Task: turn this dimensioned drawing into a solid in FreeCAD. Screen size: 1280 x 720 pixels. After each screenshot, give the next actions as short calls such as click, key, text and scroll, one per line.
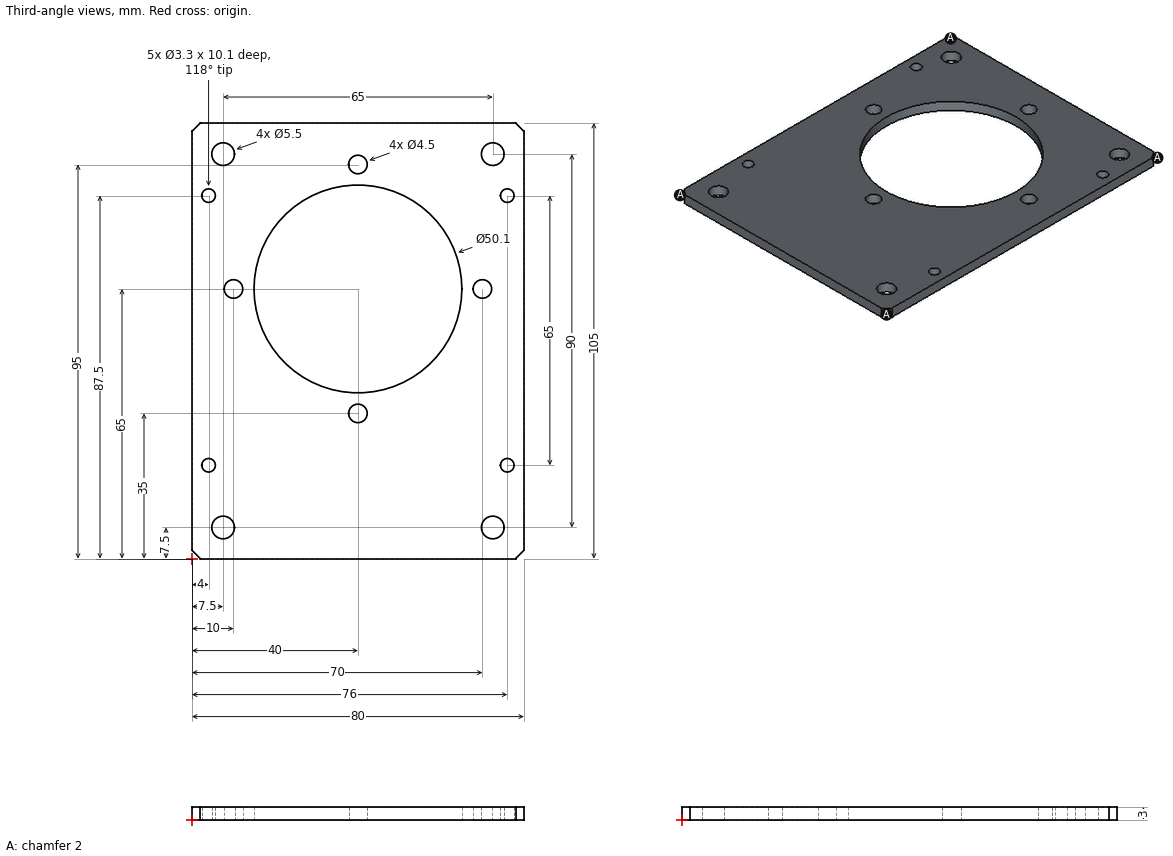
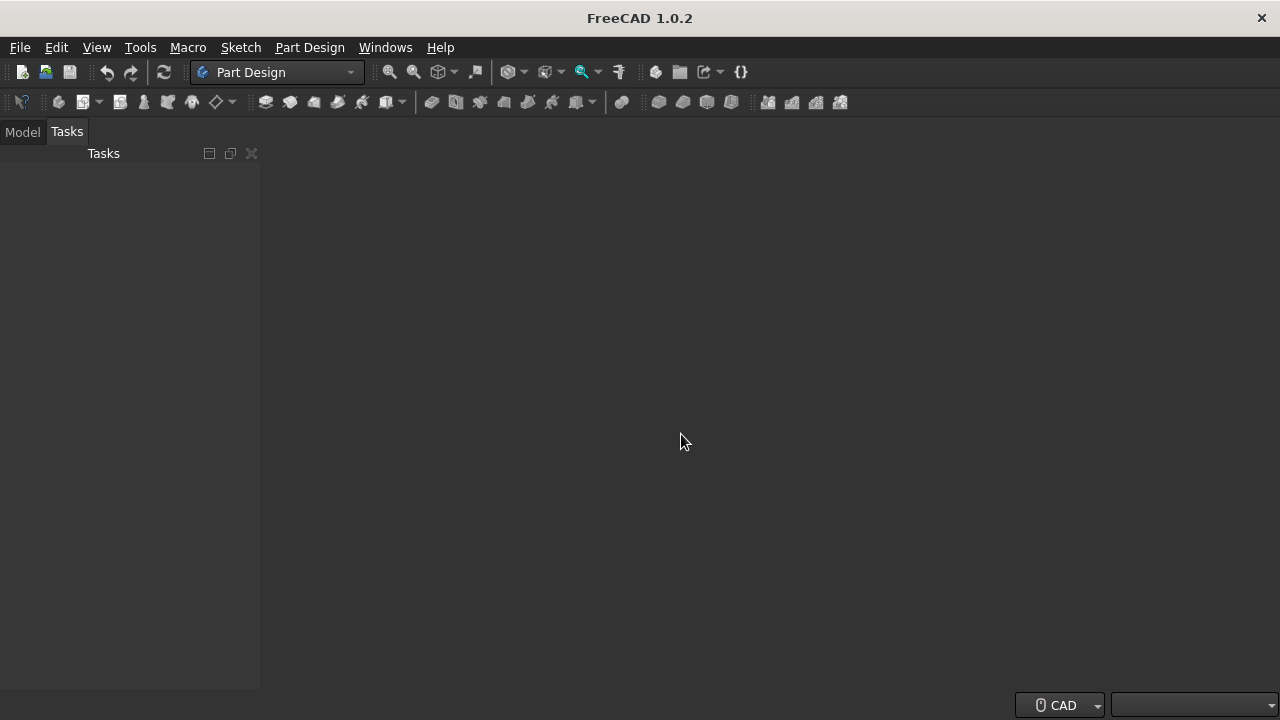
key(ctrl+n)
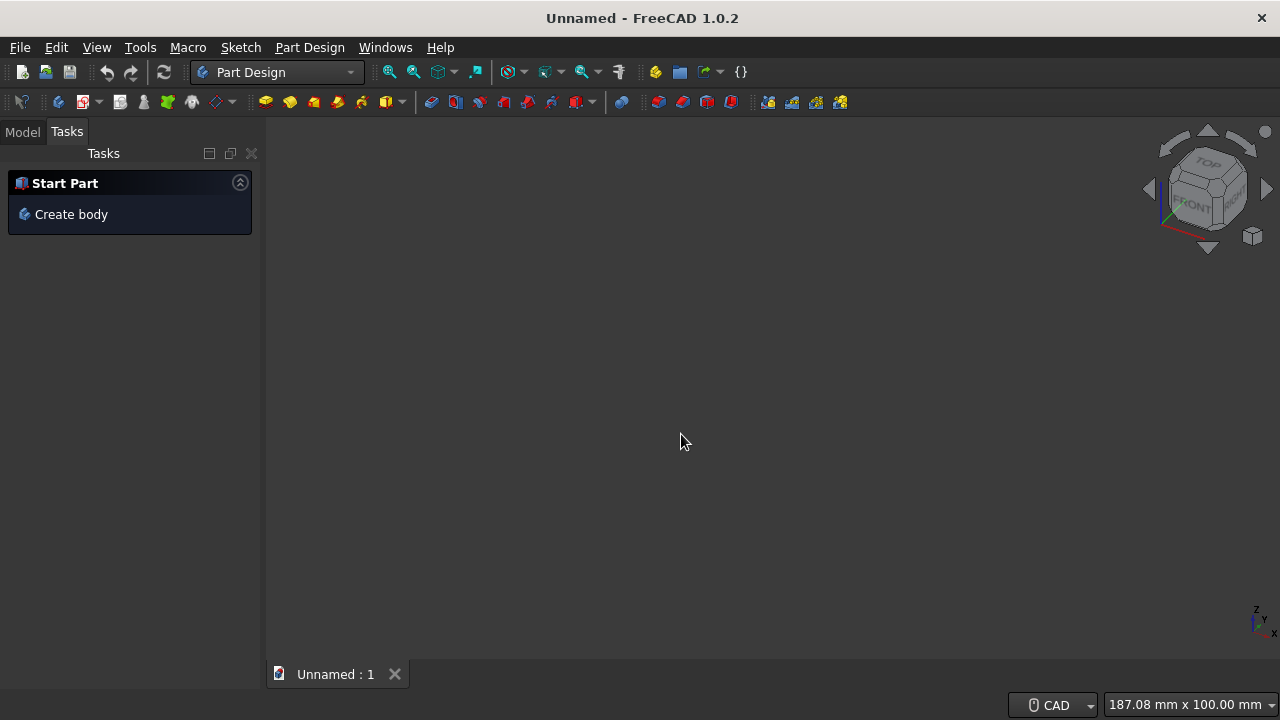
click(84, 102)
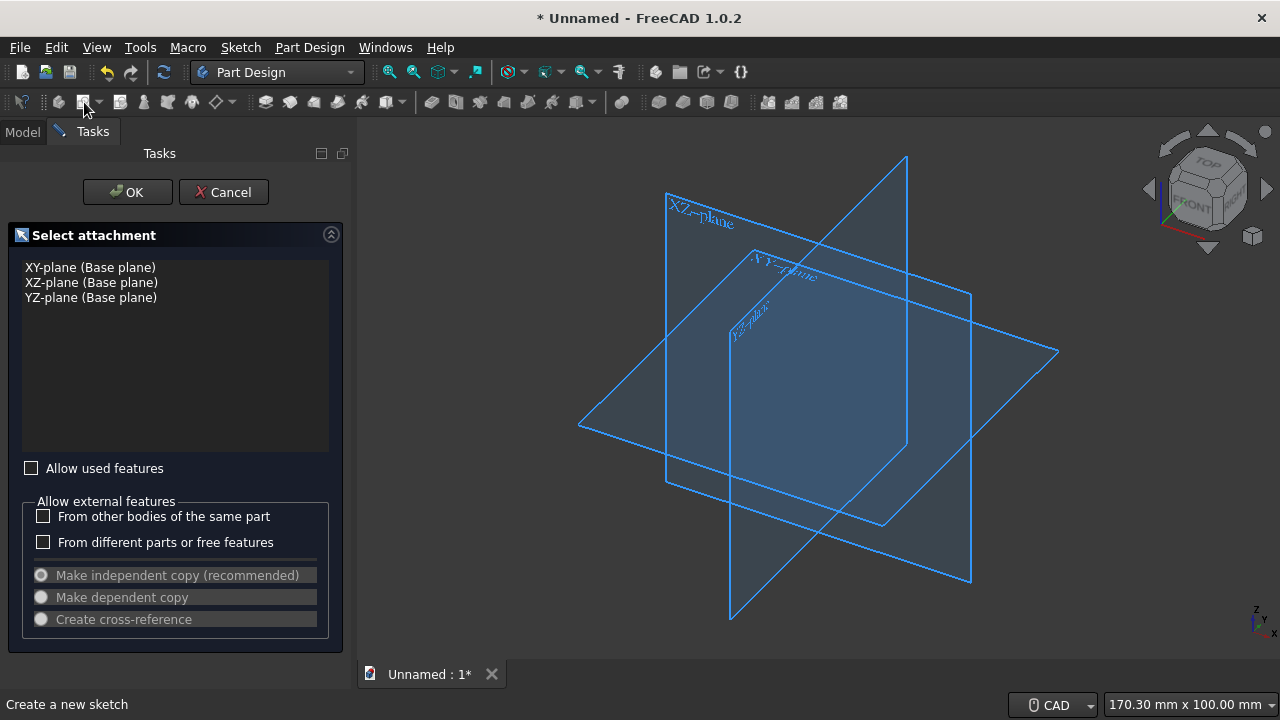
click(82, 268)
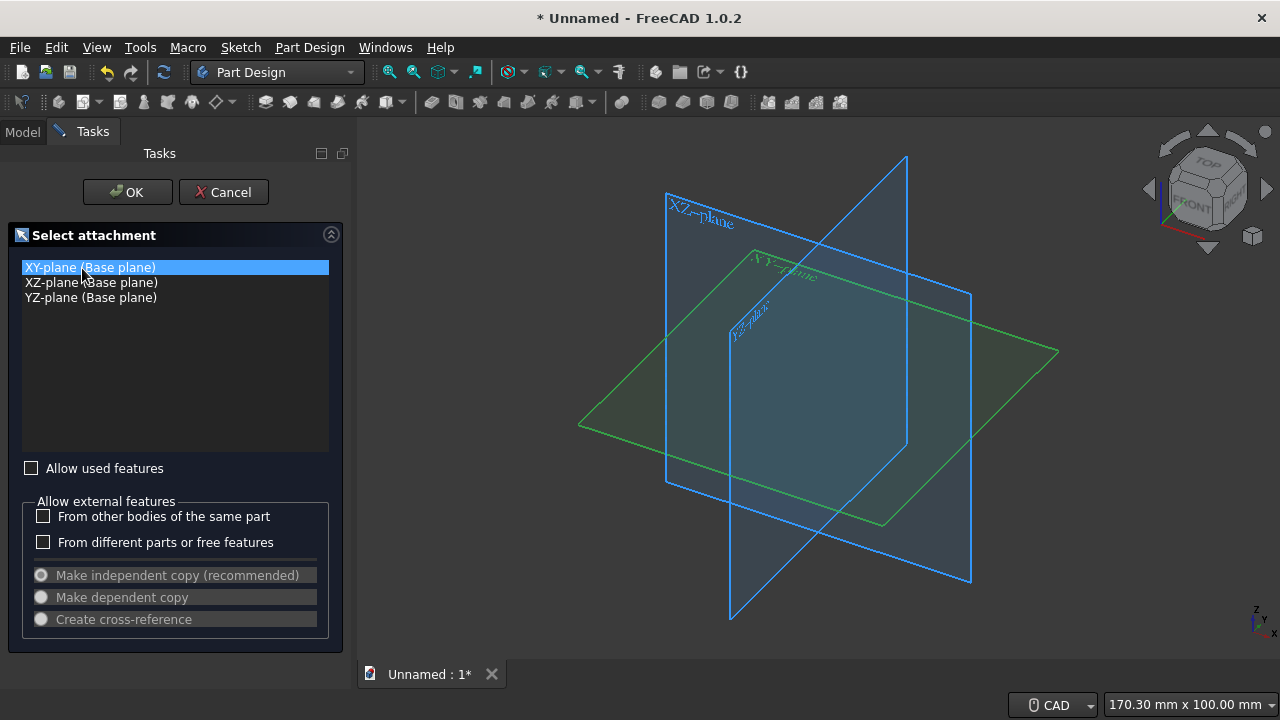
click(128, 192)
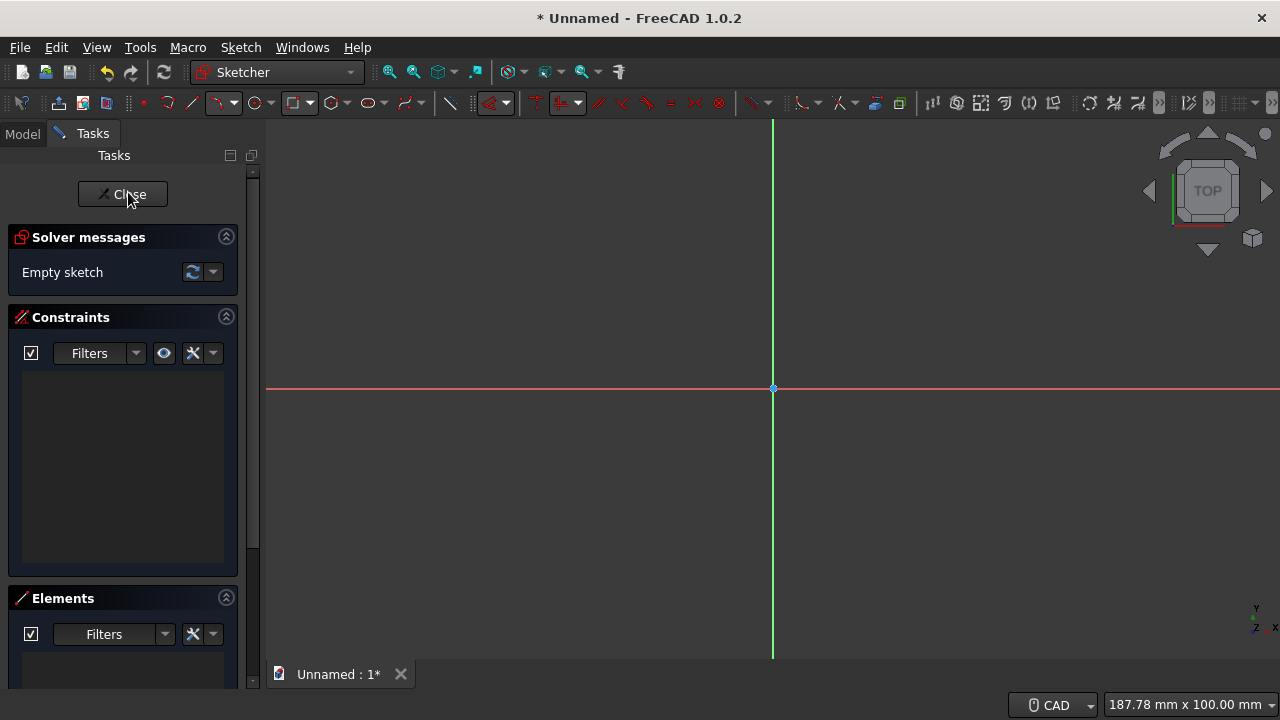
scroll(358, 631, down, 3)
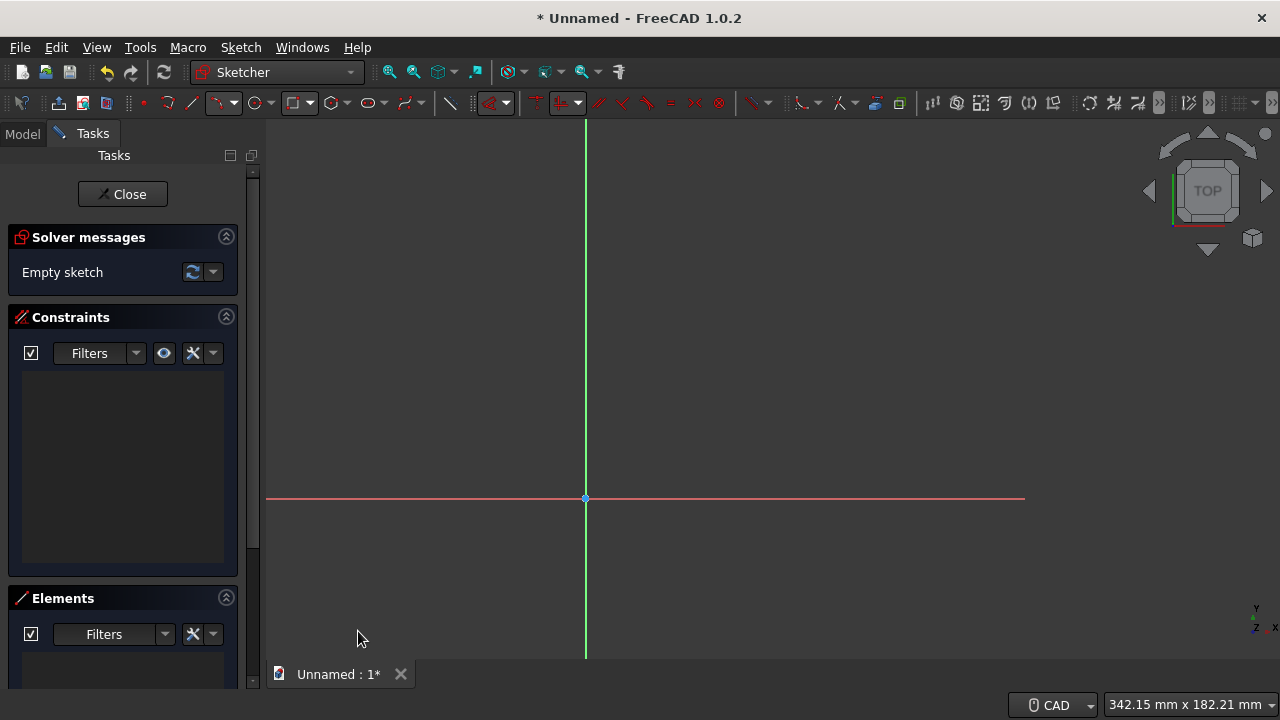
click(294, 104)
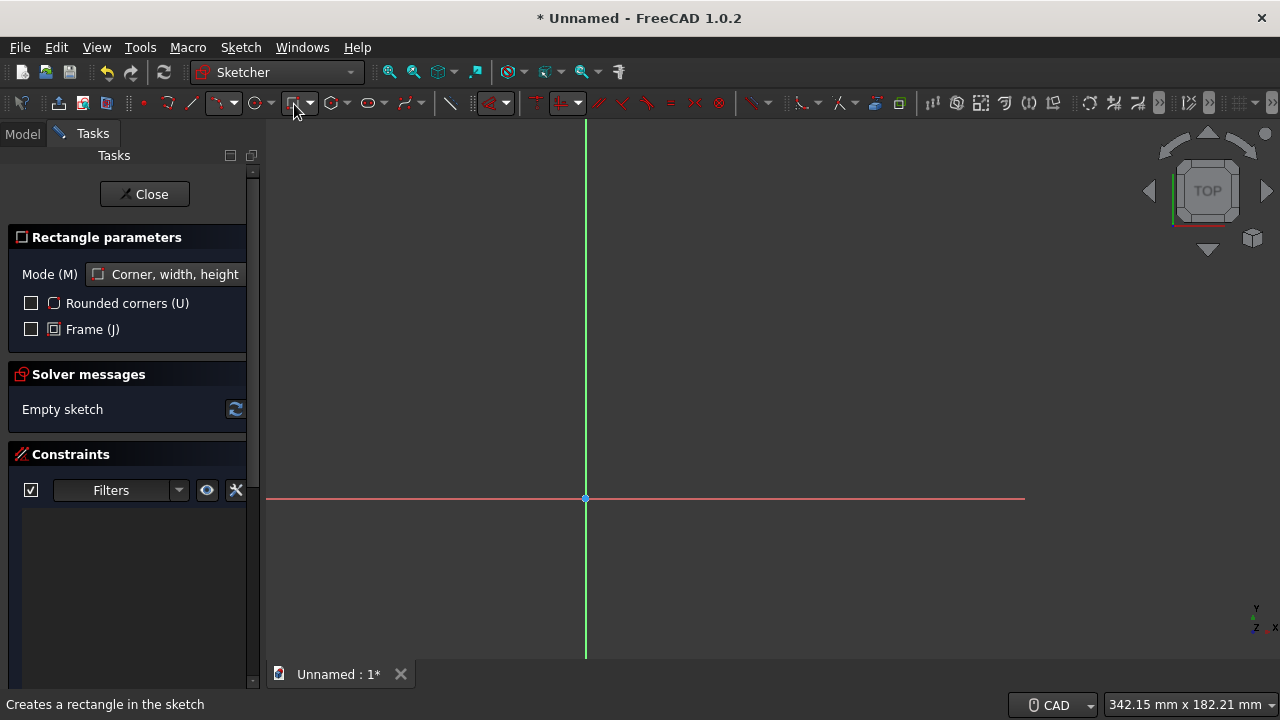
click(586, 499)
move(823, 187)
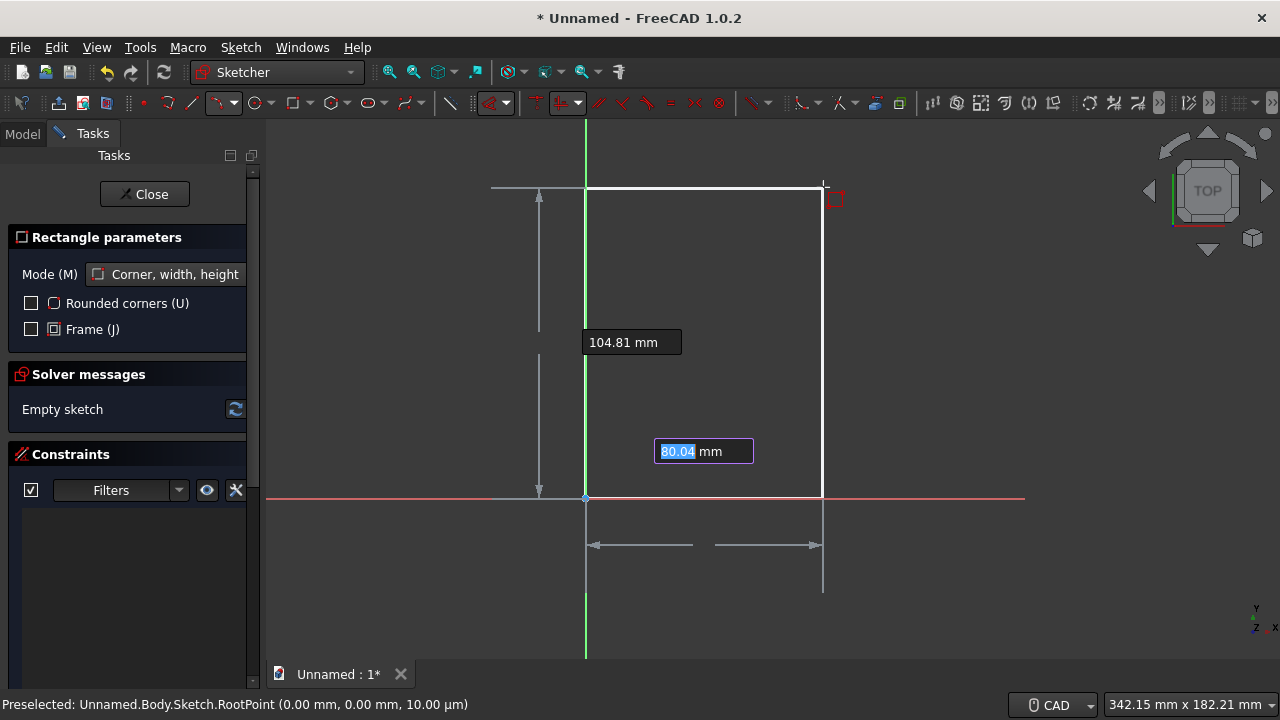
text(80)
key(Tab)
text(105)
key(Return)
key(Escape)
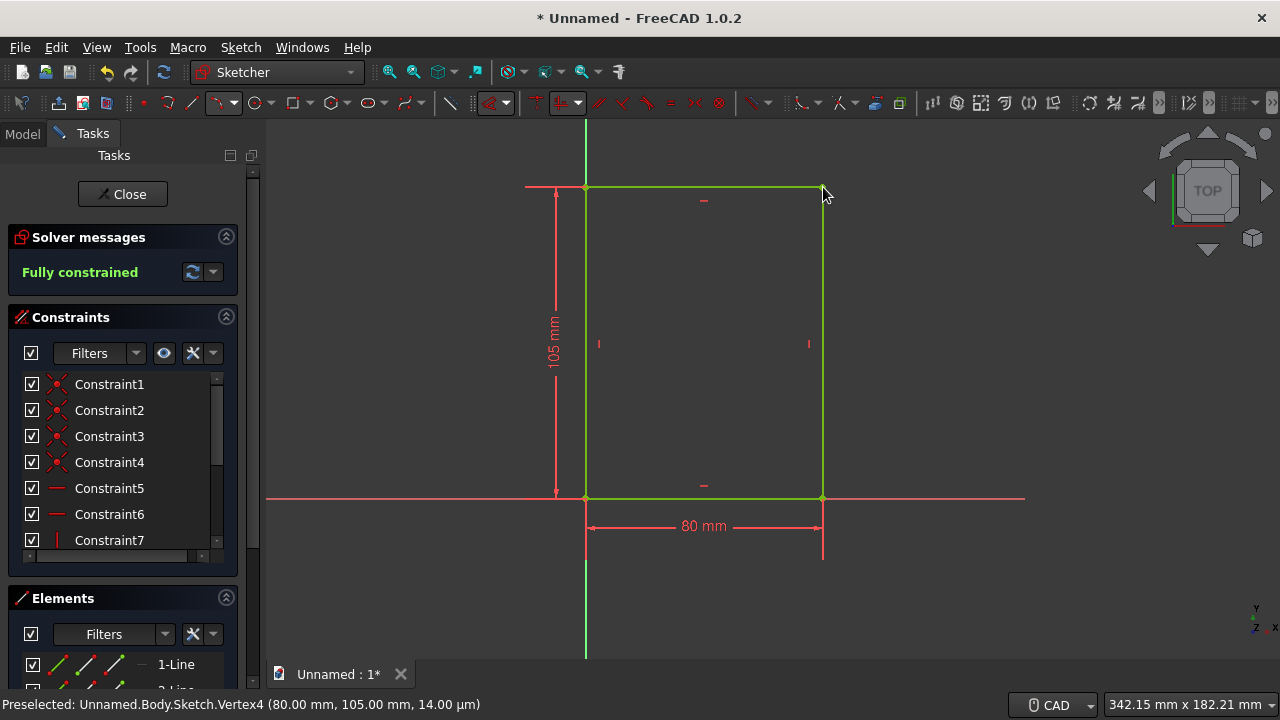
click(123, 194)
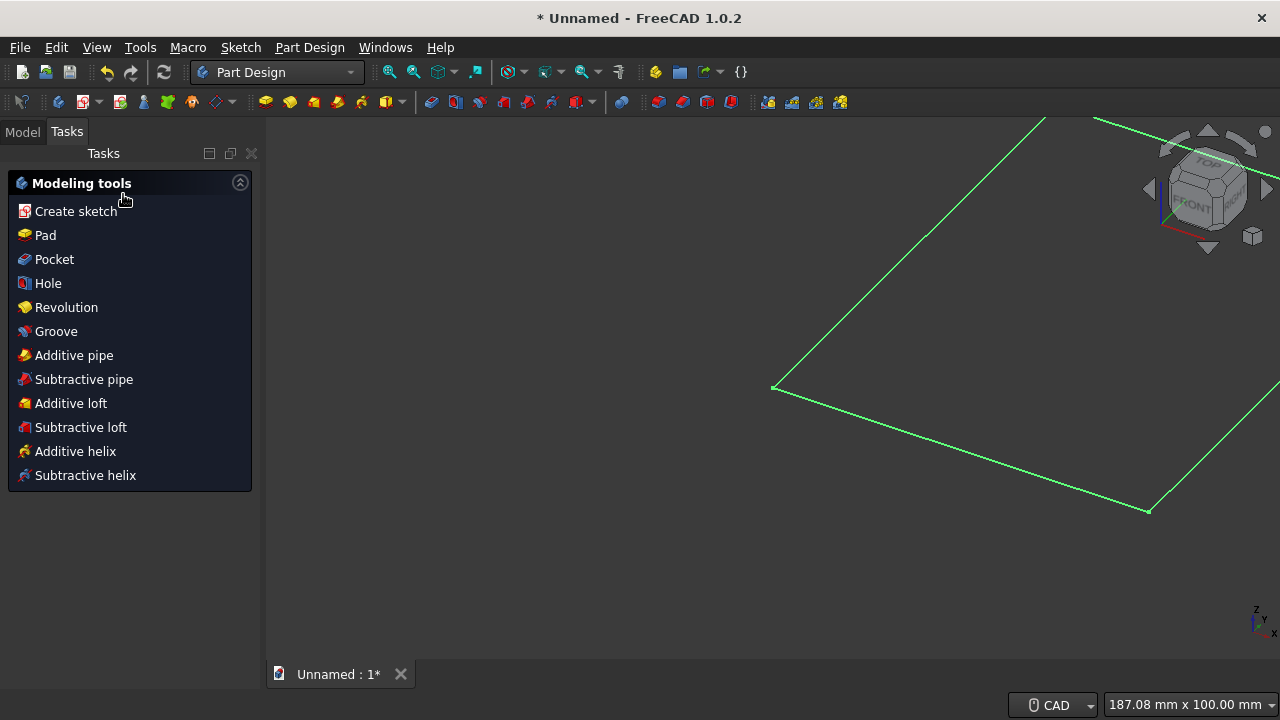
click(266, 102)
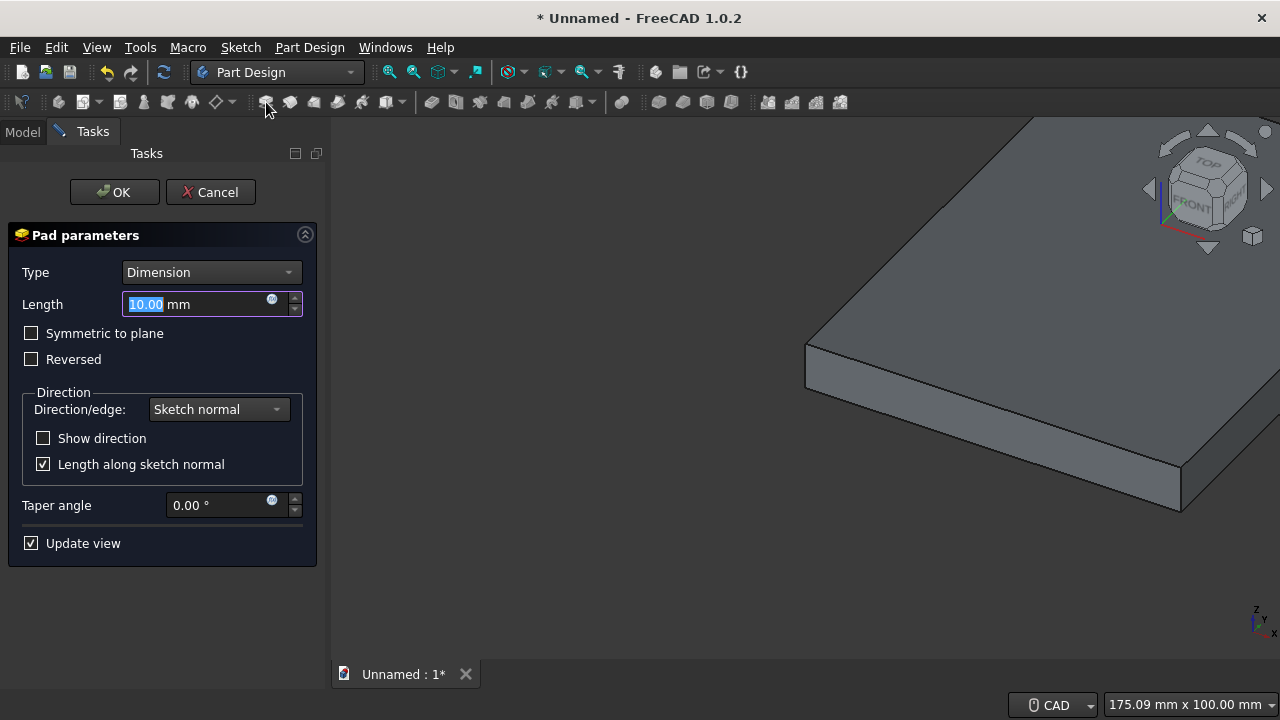
text(3)
key(Tab)